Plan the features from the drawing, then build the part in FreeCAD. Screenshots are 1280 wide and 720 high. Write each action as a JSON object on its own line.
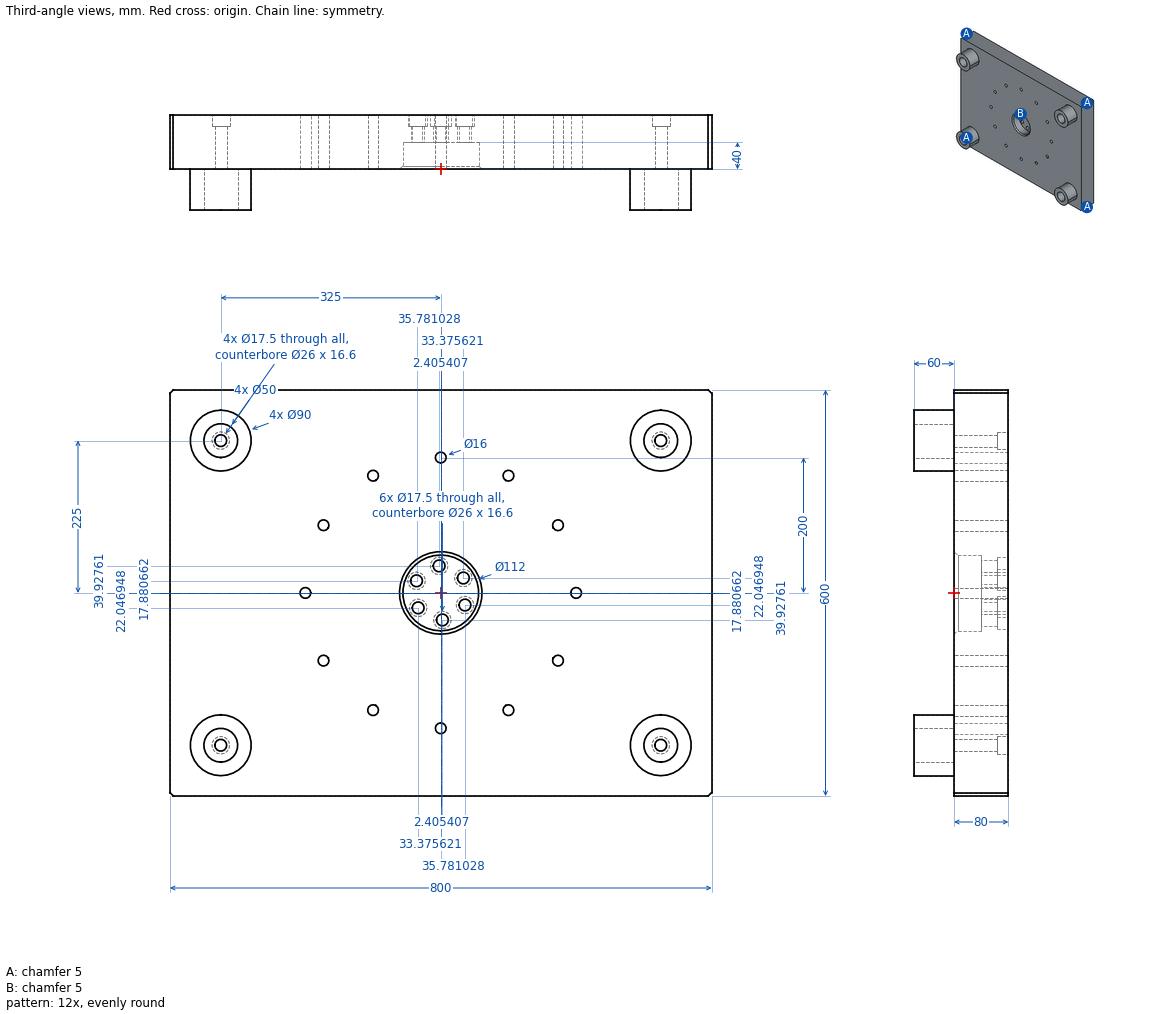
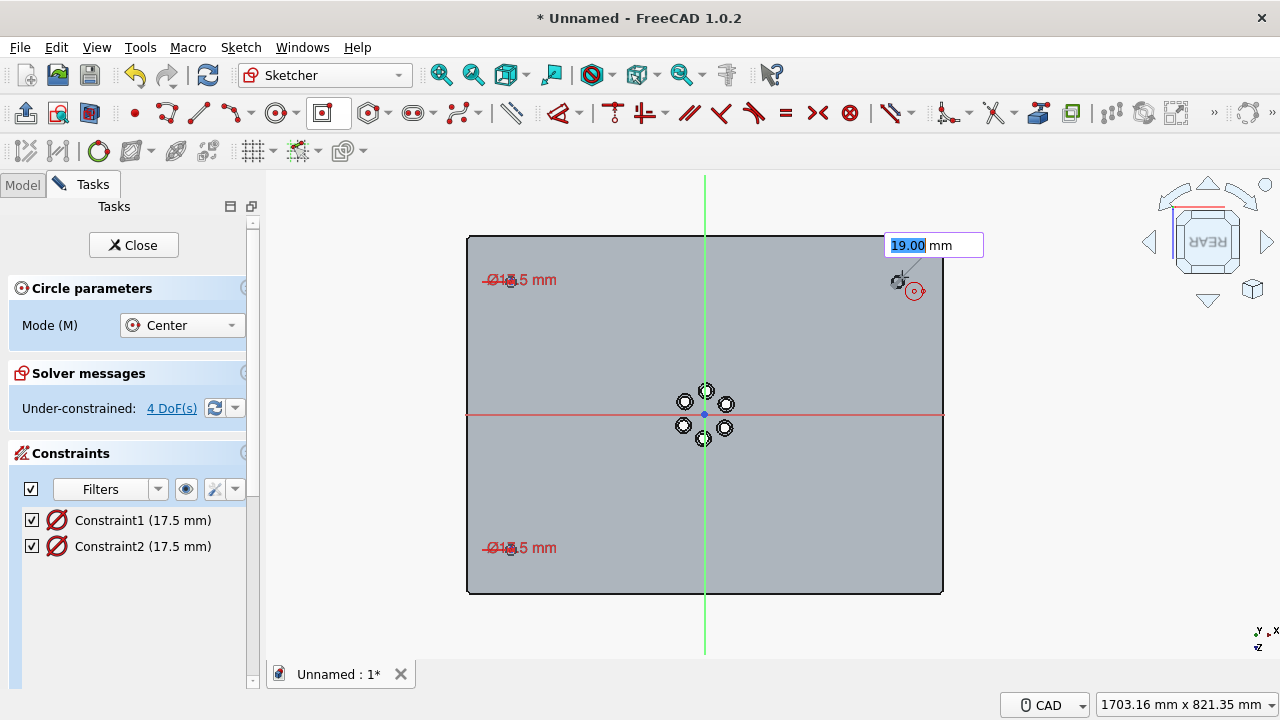
{"action": "type", "text": "17.5"}
{"action": "key", "text": "Return"}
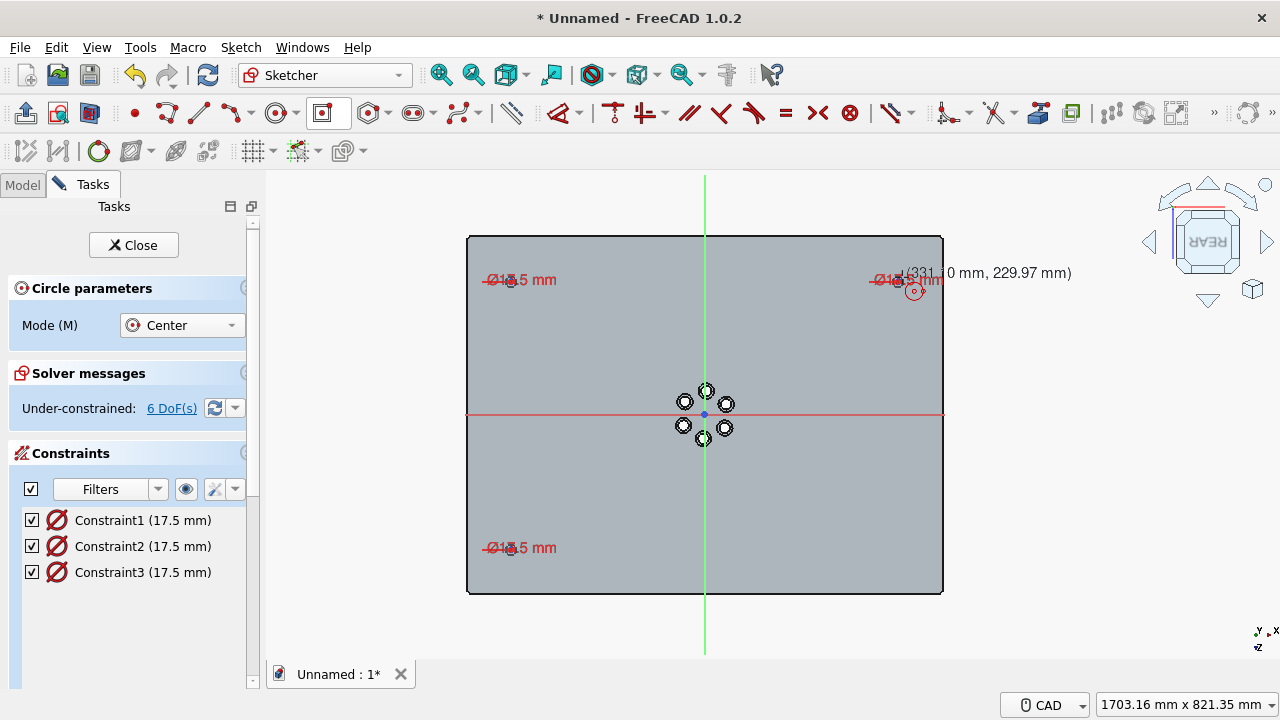
{"action": "scroll", "coordinate": [898, 549], "scroll_direction": "up", "scroll_amount": 8}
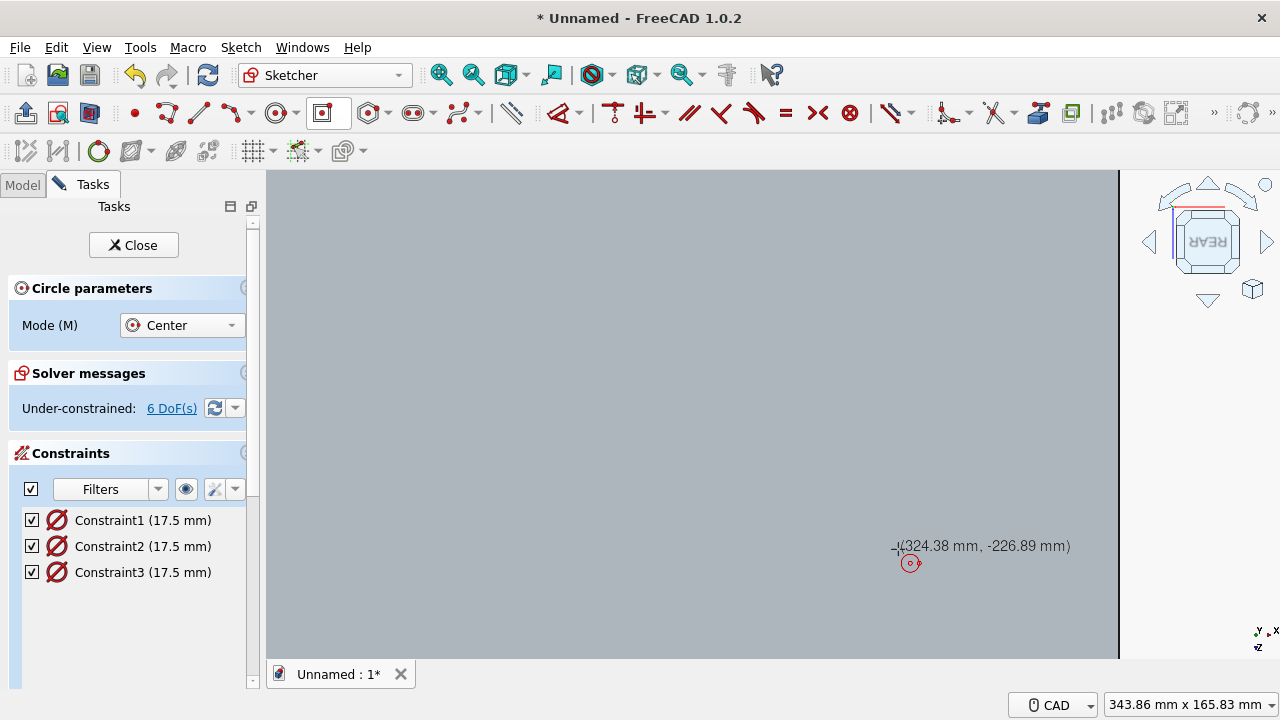
{"action": "scroll", "coordinate": [898, 549], "scroll_direction": "down", "scroll_amount": 8}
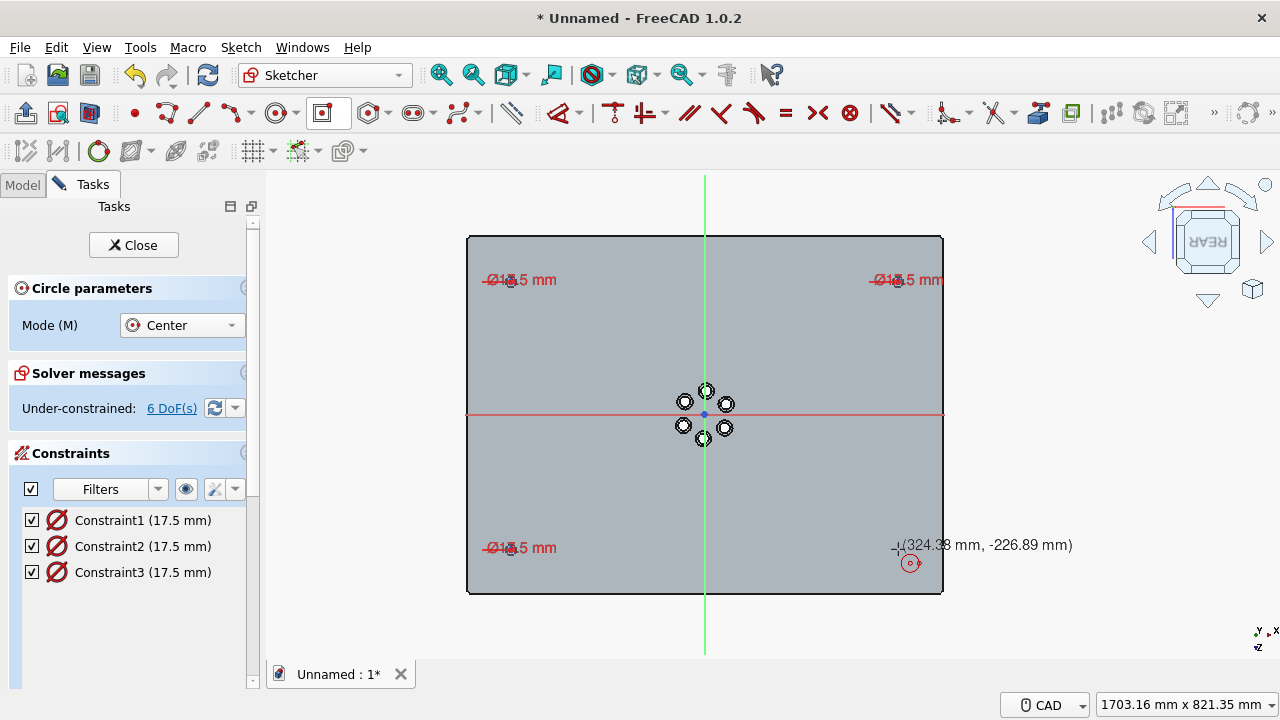
{"action": "left_click", "coordinate": [898, 549]}
{"action": "mouse_move", "coordinate": [902, 545]}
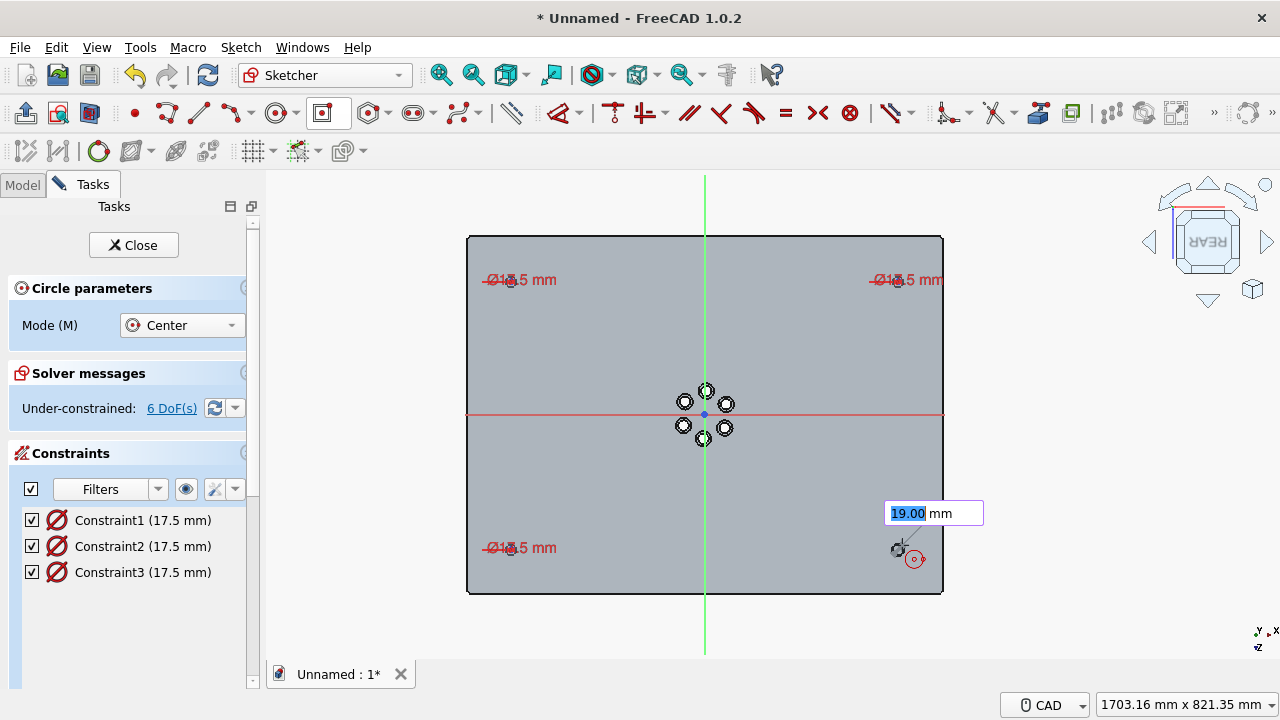
{"action": "type", "text": "17.5"}
{"action": "key", "text": "Return"}
{"action": "key", "text": "Escape"}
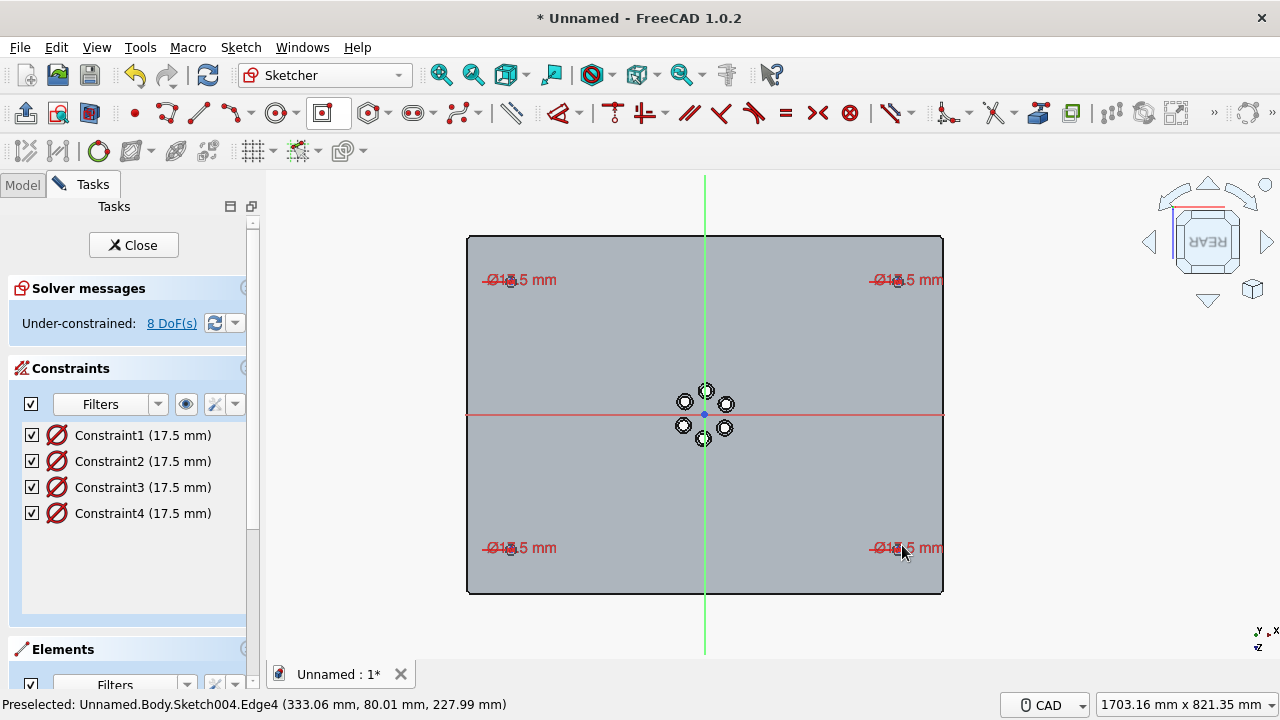
{"action": "left_click", "coordinate": [511, 550]}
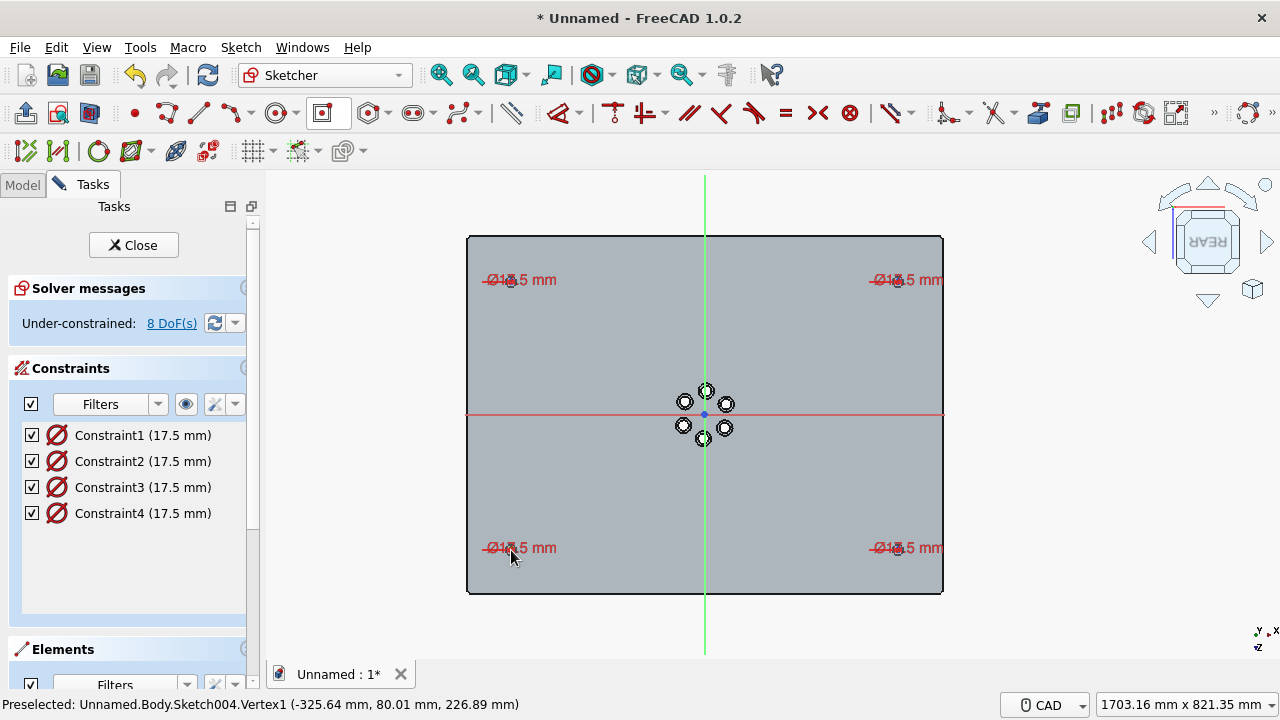
{"action": "left_click", "coordinate": [511, 282]}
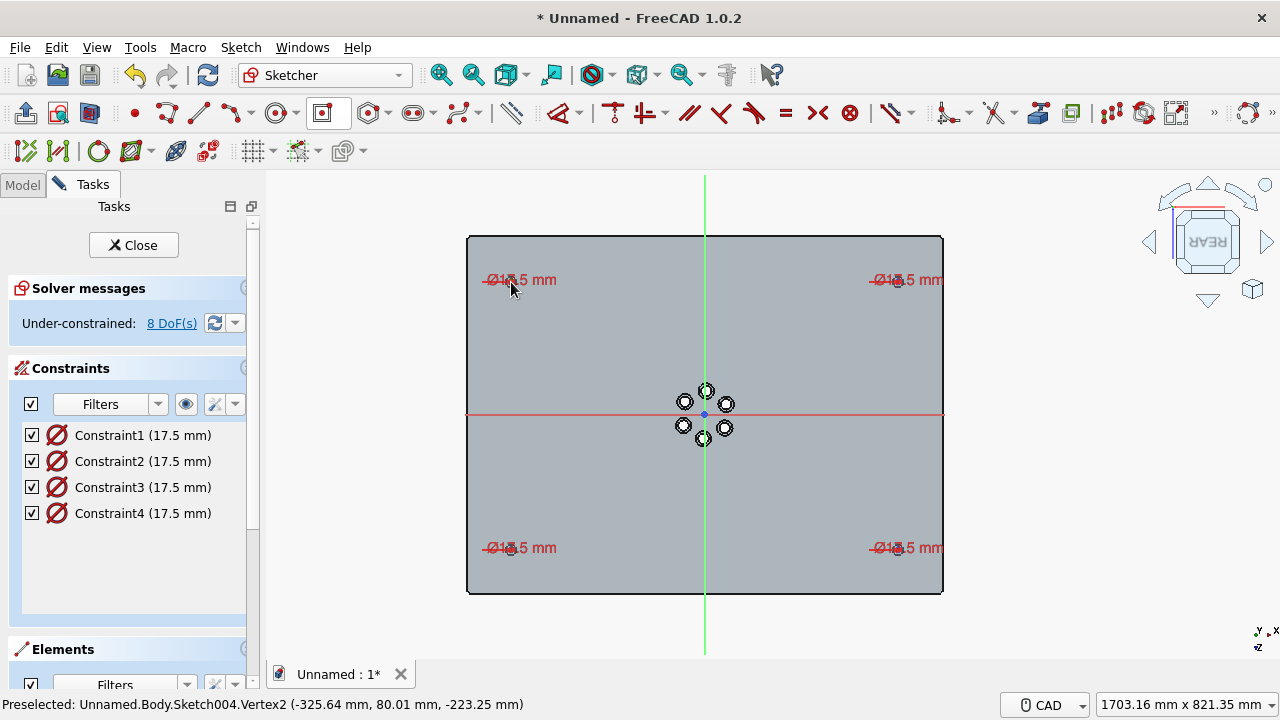
{"action": "left_click", "coordinate": [470, 415]}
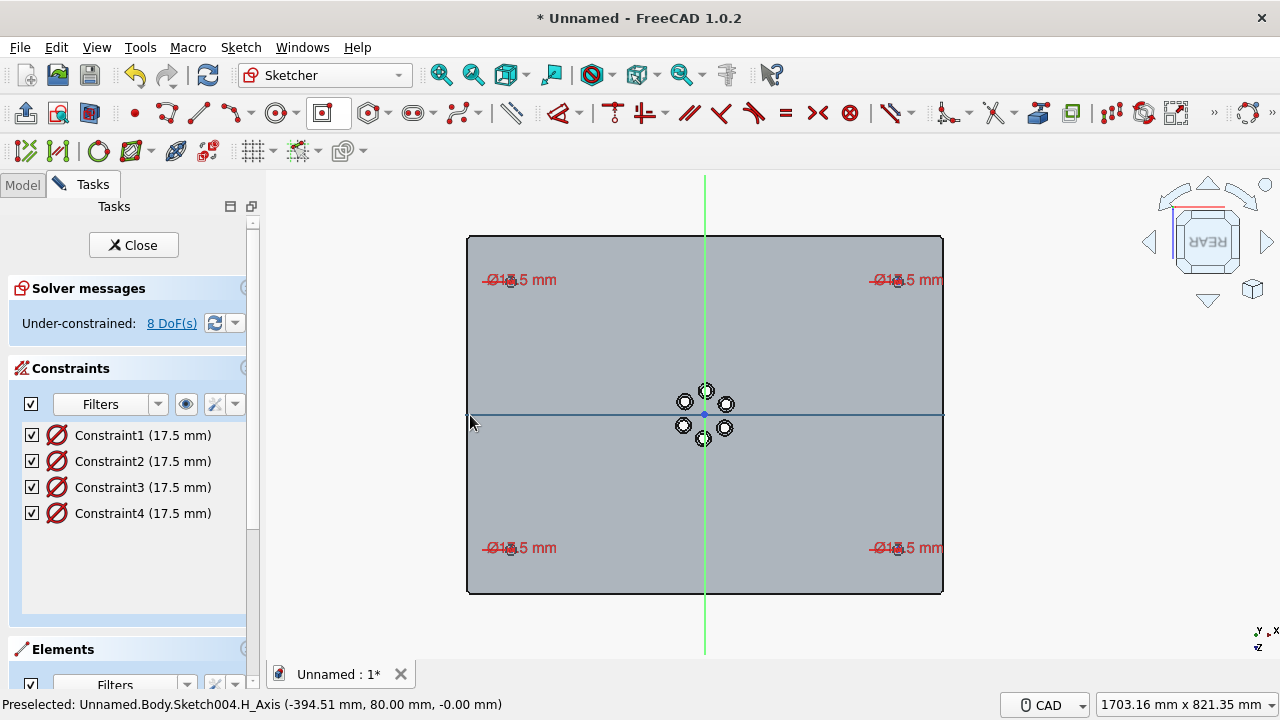
{"action": "key", "text": "s"}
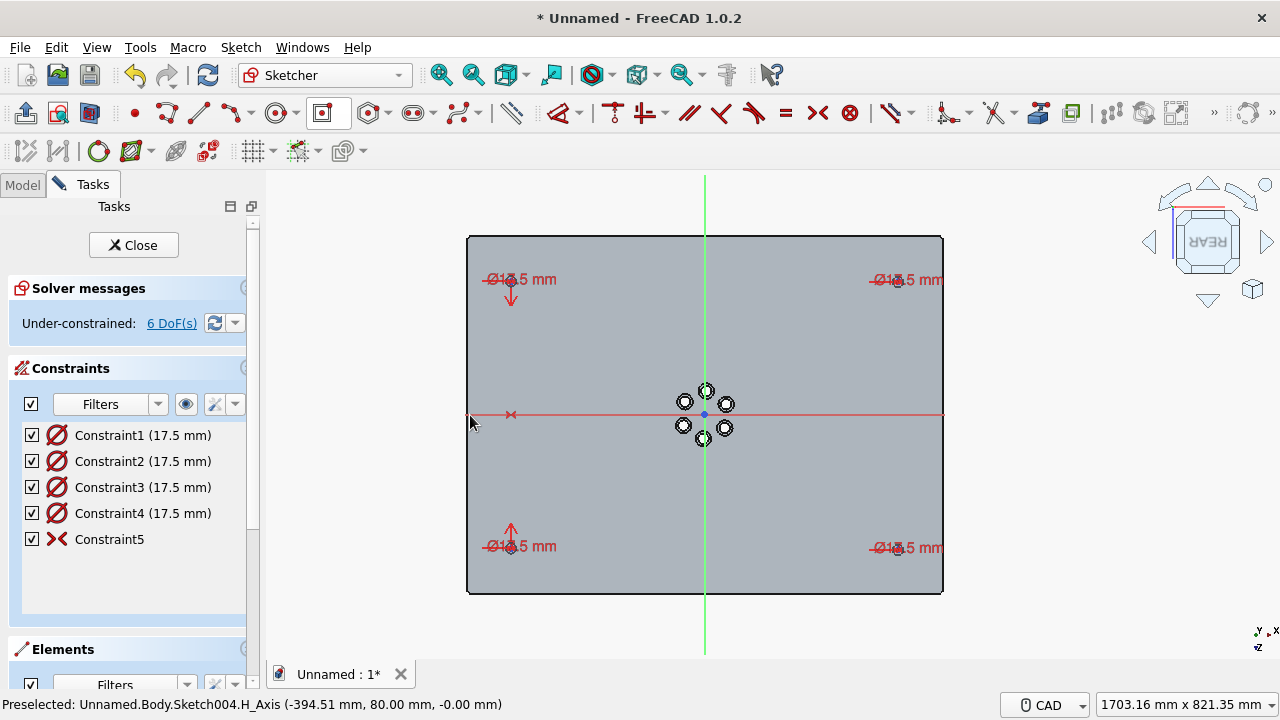
{"action": "left_click", "coordinate": [511, 281]}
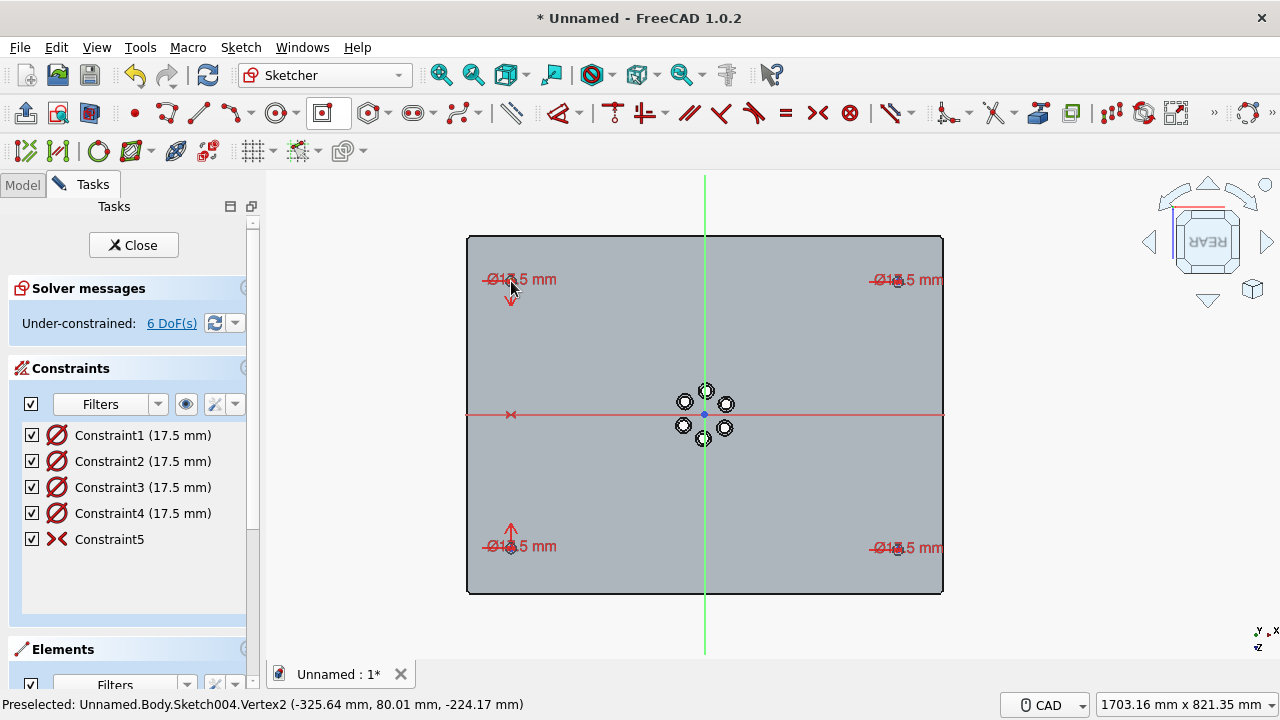
{"action": "left_click", "coordinate": [898, 282]}